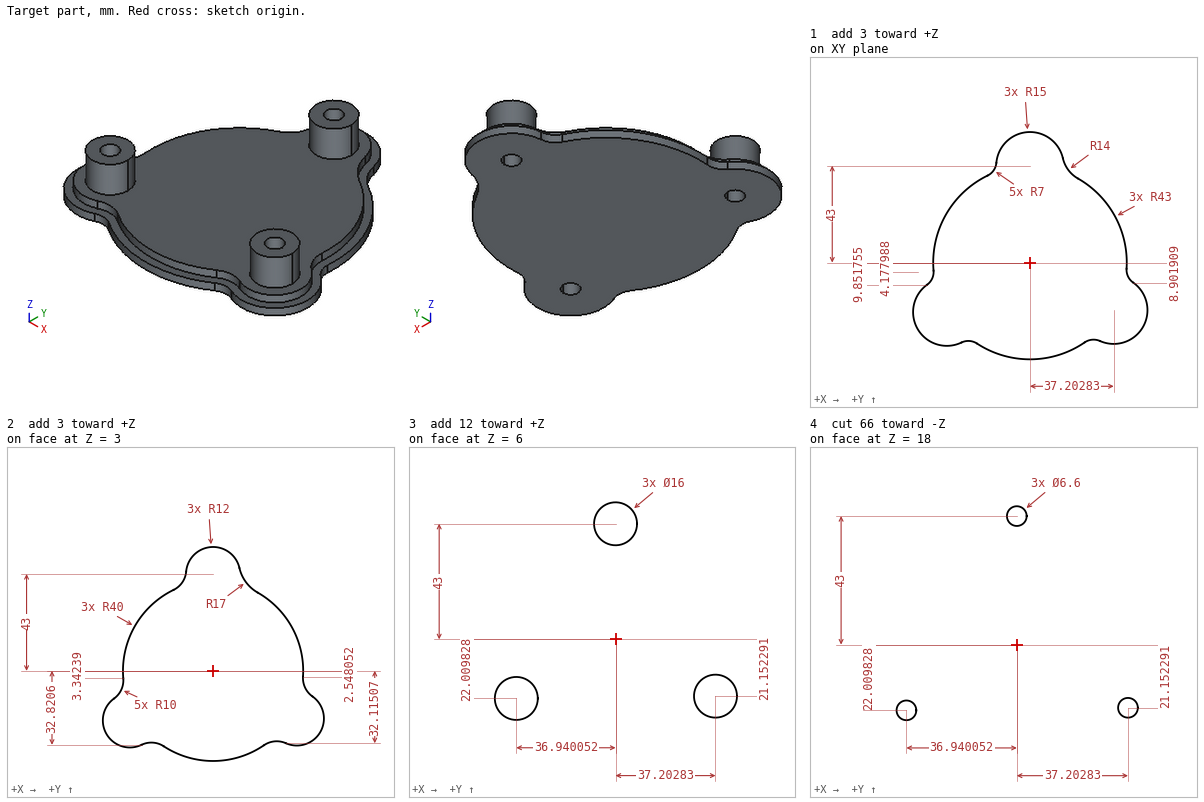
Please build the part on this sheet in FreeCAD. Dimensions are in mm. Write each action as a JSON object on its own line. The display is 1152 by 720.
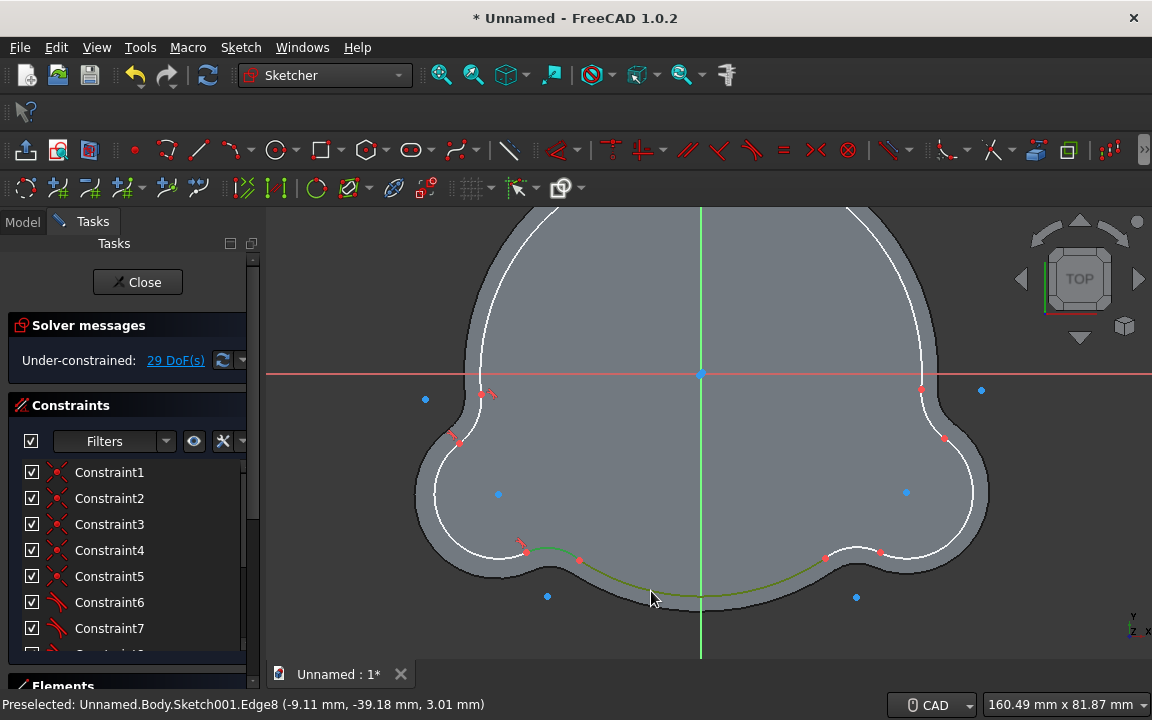
{"action": "left_click", "coordinate": [752, 150]}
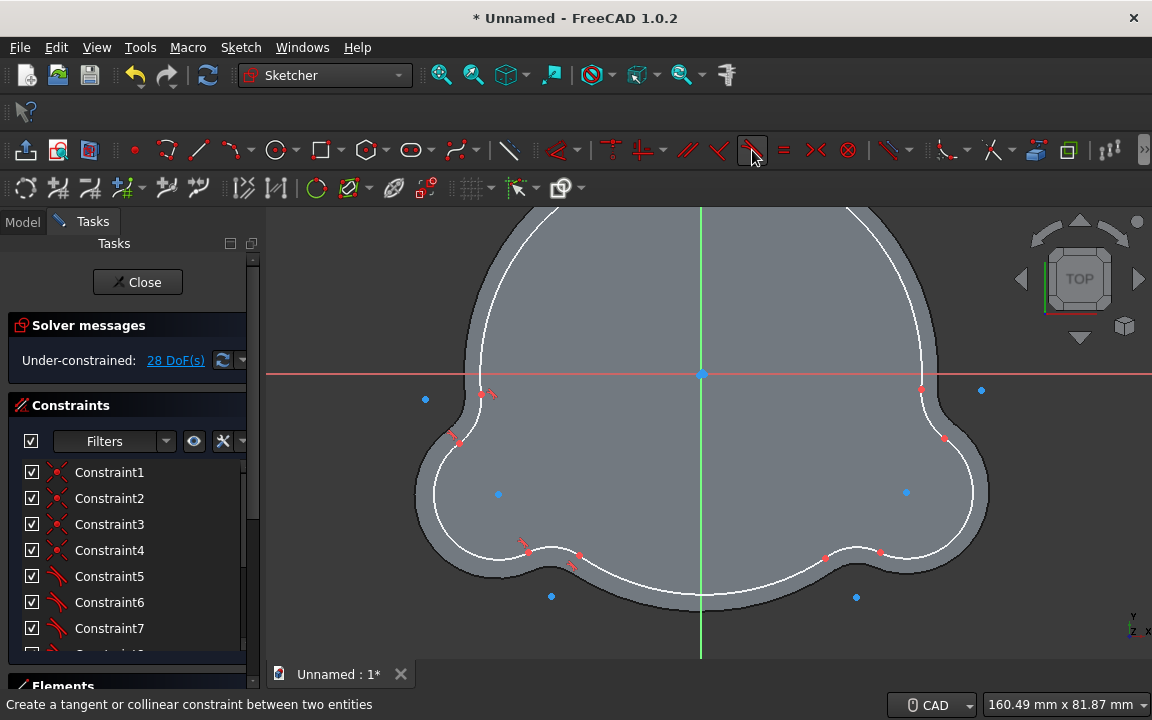
{"action": "left_click", "coordinate": [650, 588]}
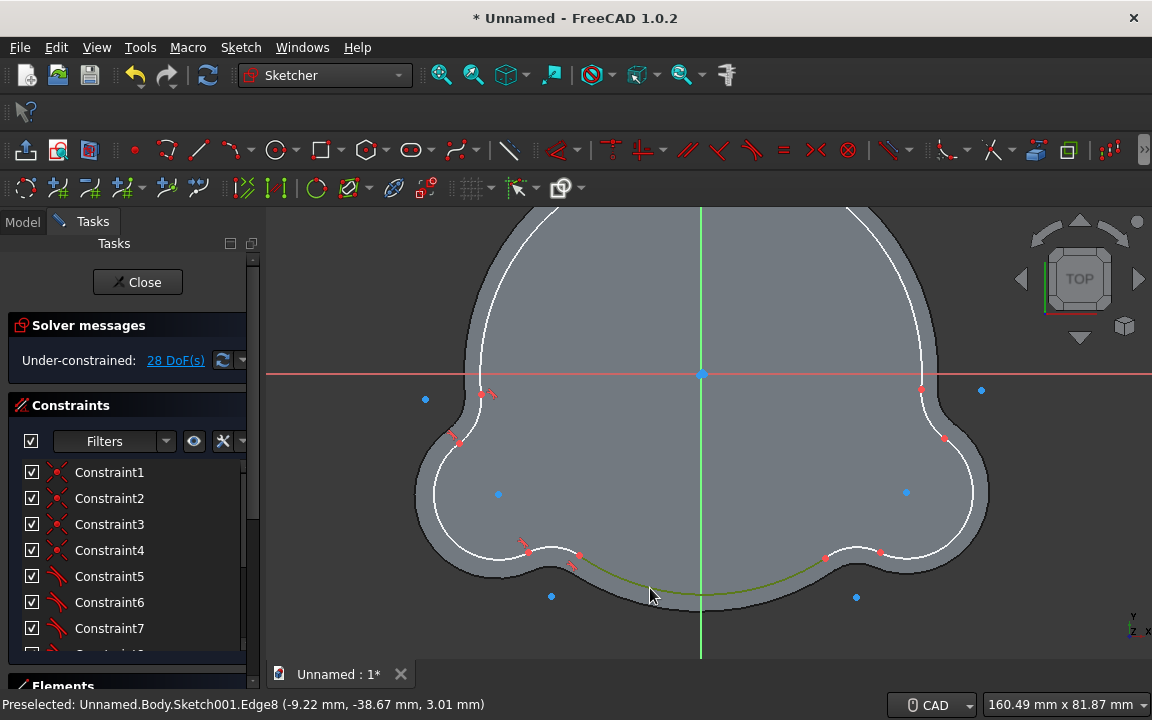
{"action": "left_click", "coordinate": [863, 548]}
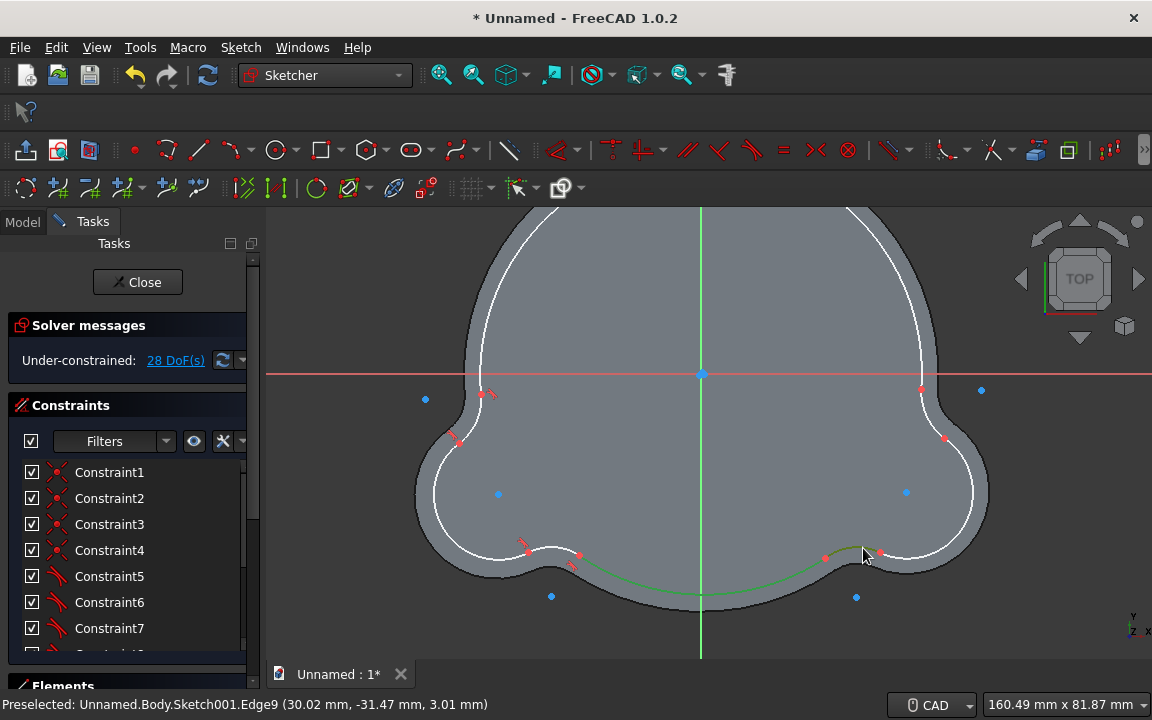
{"action": "left_click", "coordinate": [752, 150]}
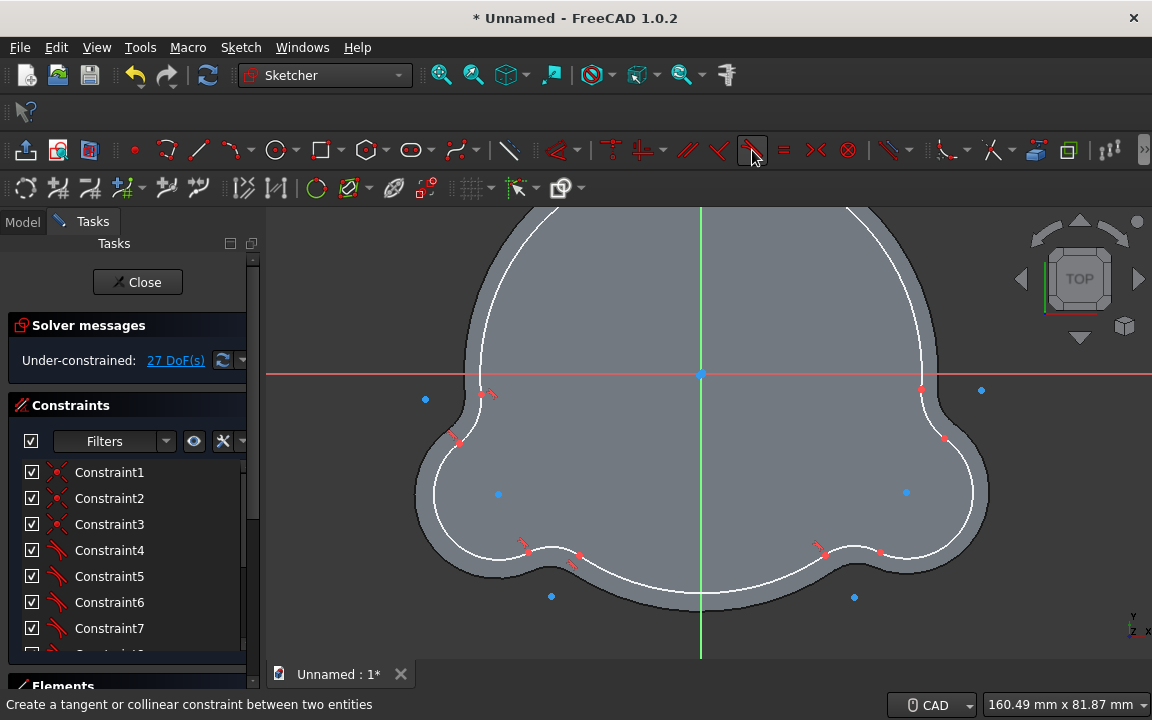
{"action": "left_click", "coordinate": [864, 547]}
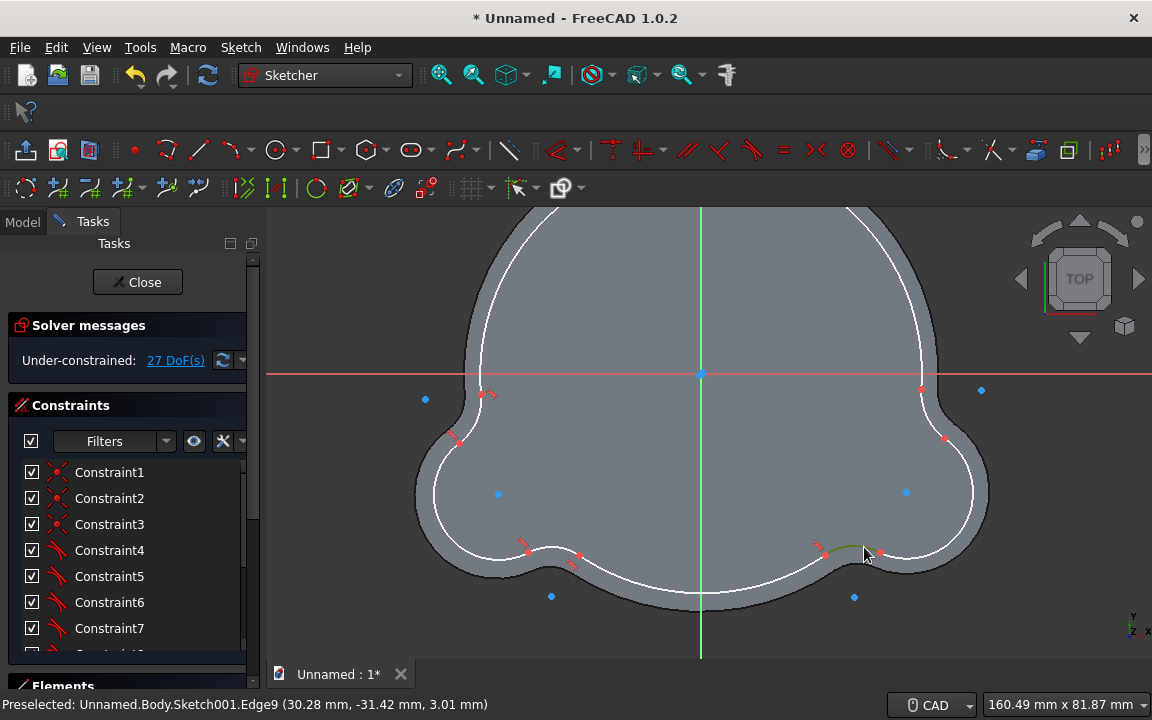
{"action": "left_click", "coordinate": [937, 552]}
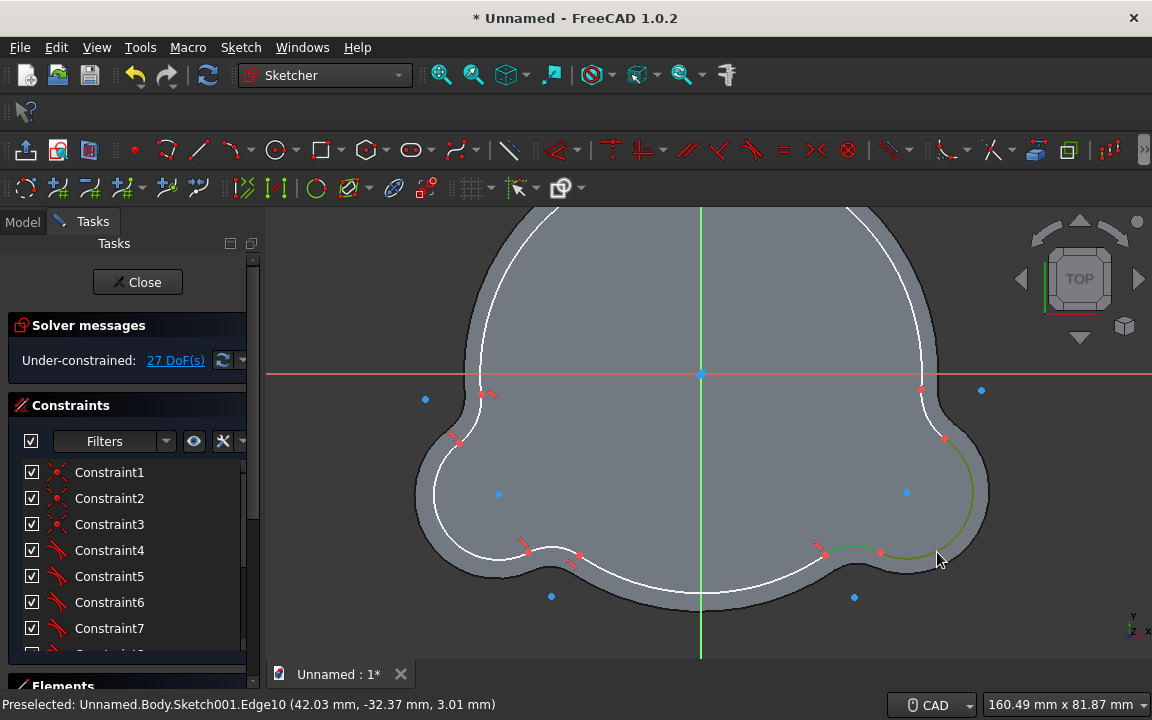
{"action": "left_click", "coordinate": [752, 150]}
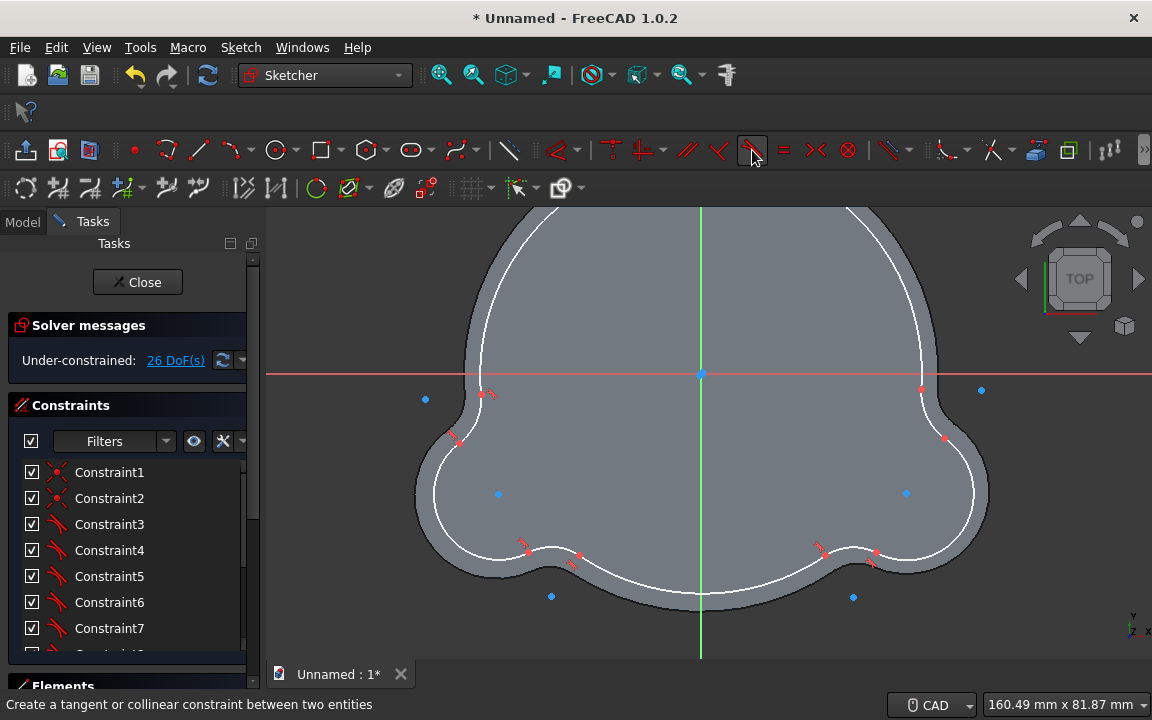
{"action": "left_click", "coordinate": [935, 554]}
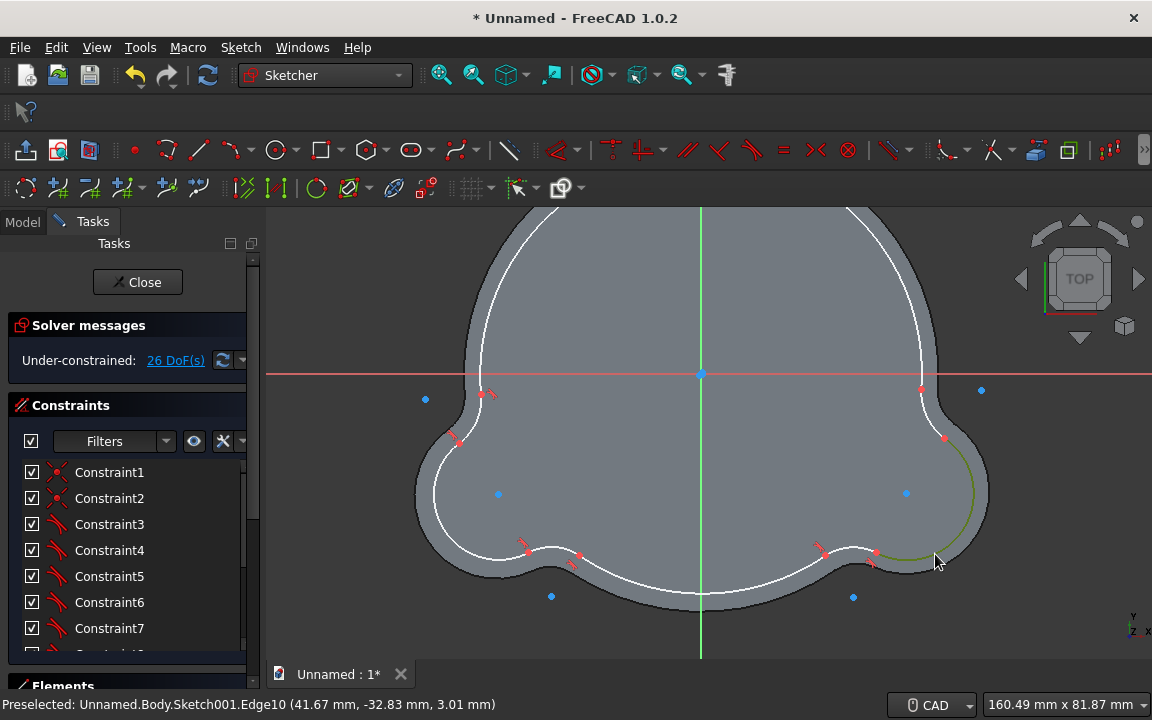
{"action": "left_click", "coordinate": [923, 406]}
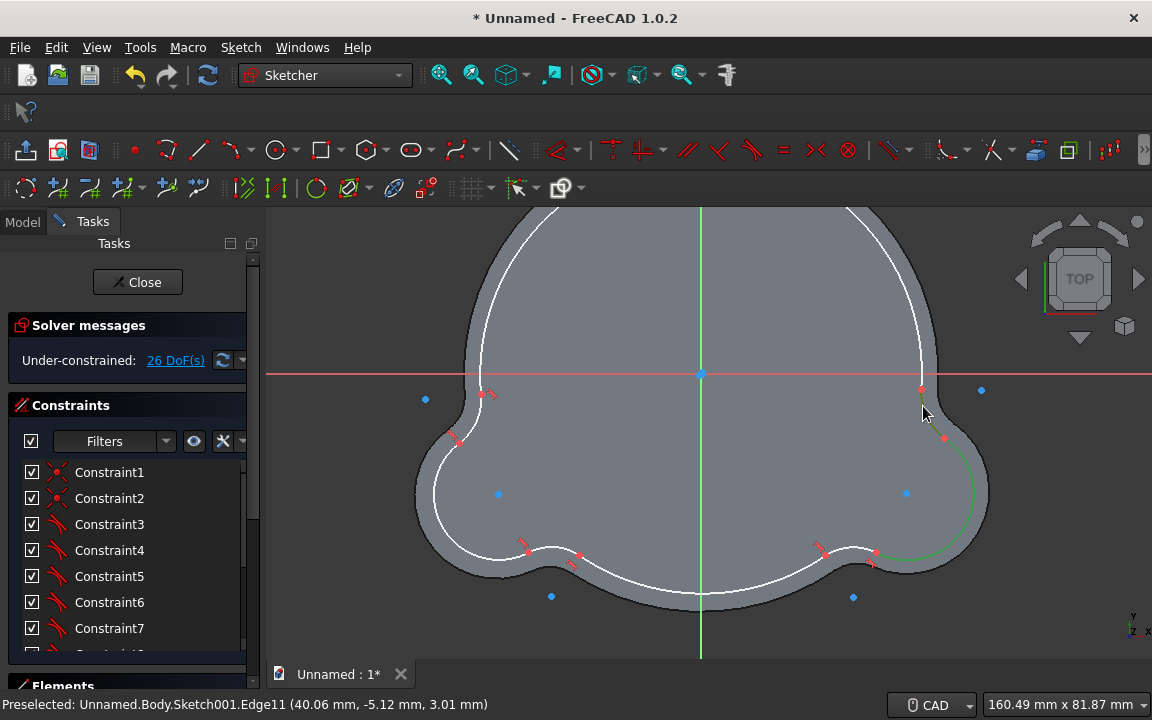
{"action": "left_click", "coordinate": [752, 150]}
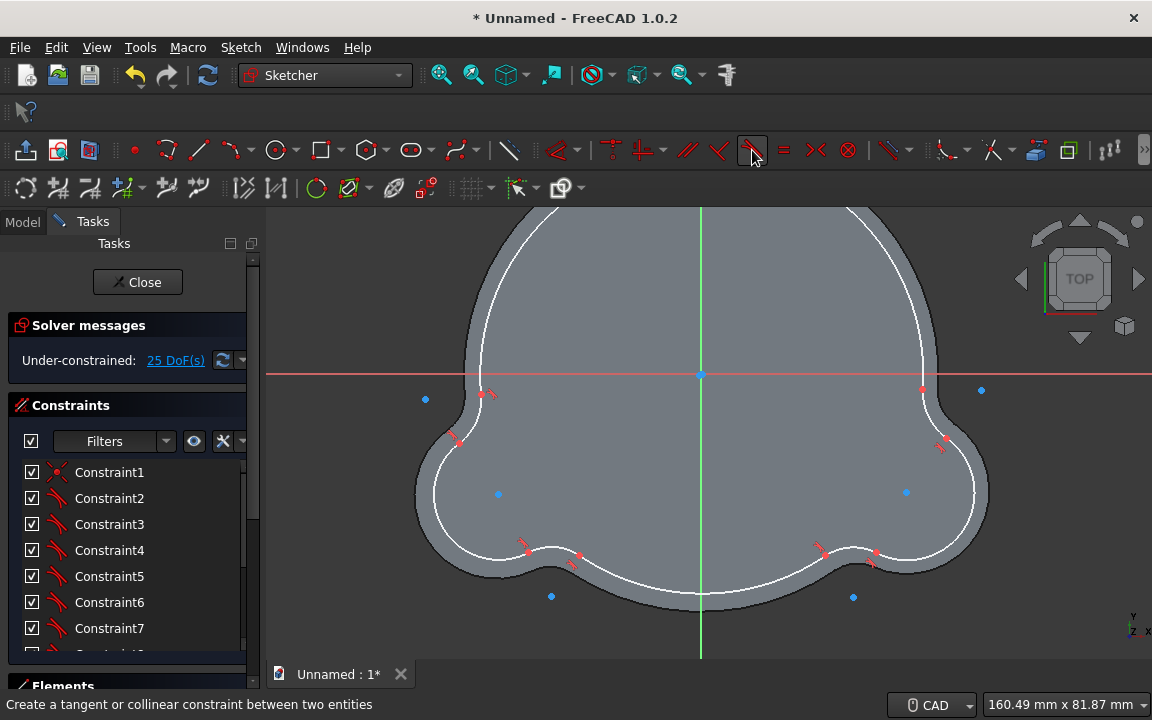
{"action": "left_click", "coordinate": [925, 406]}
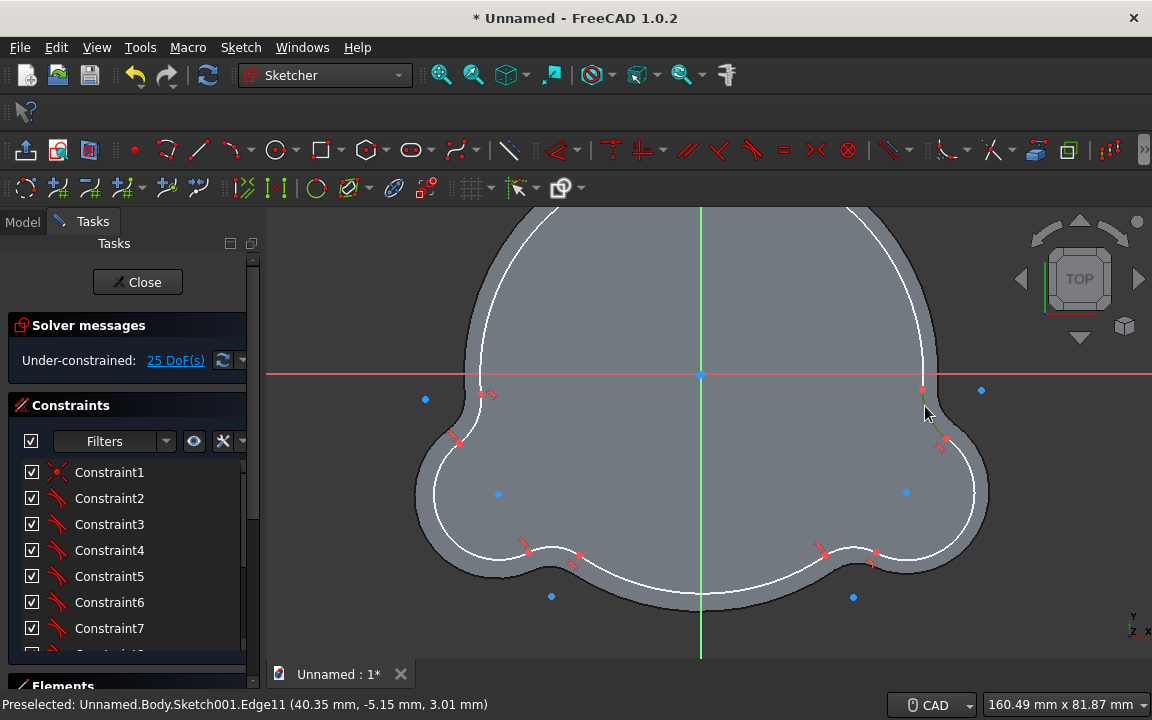
{"action": "left_click", "coordinate": [916, 317]}